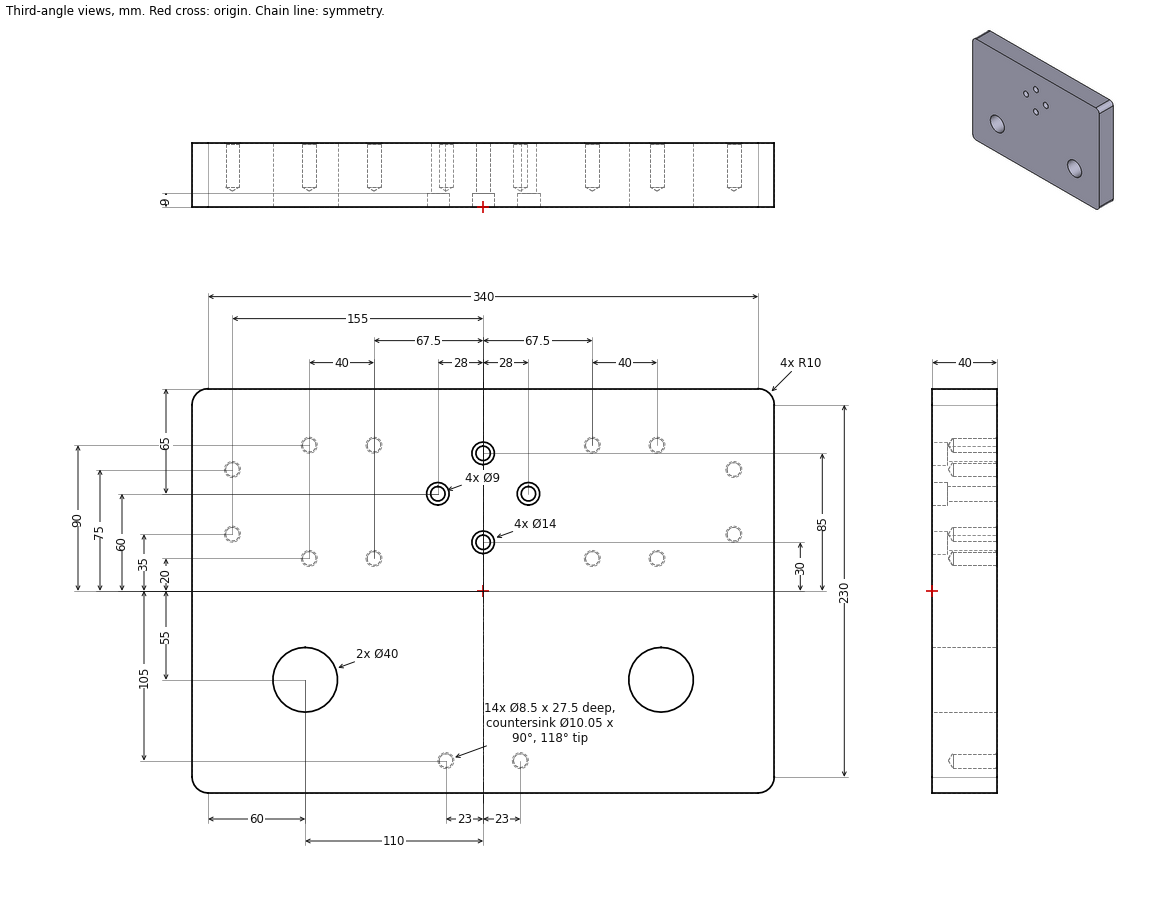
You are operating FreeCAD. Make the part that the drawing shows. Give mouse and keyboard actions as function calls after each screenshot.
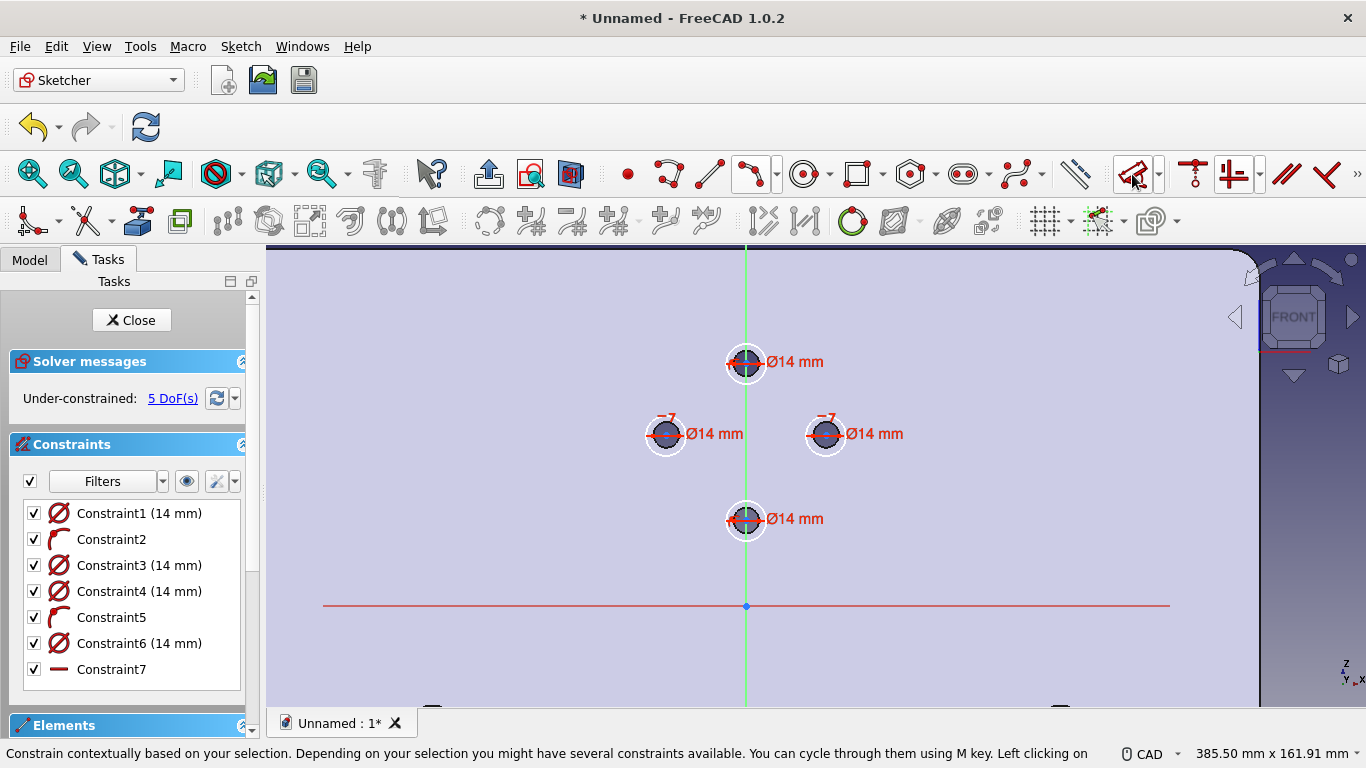
click(746, 521)
click(780, 564)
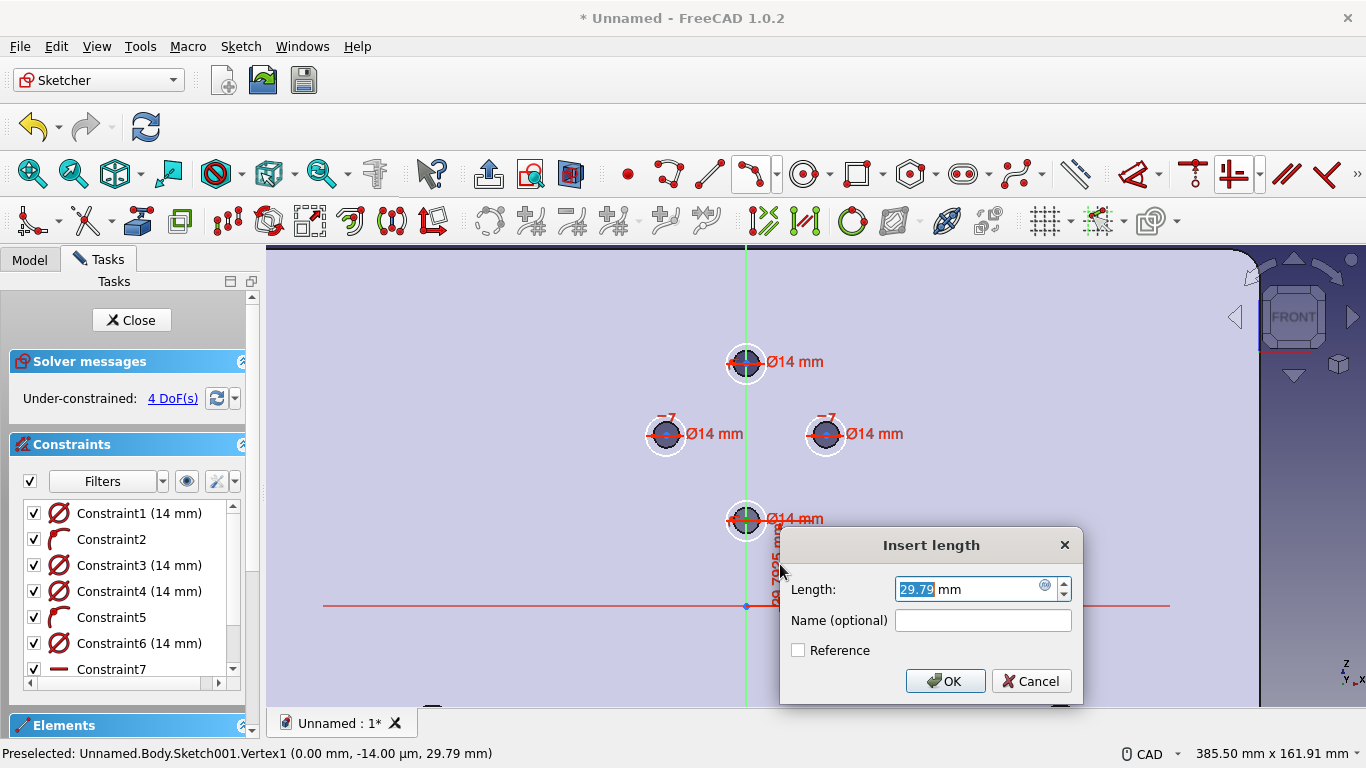
text(30)
key(Return)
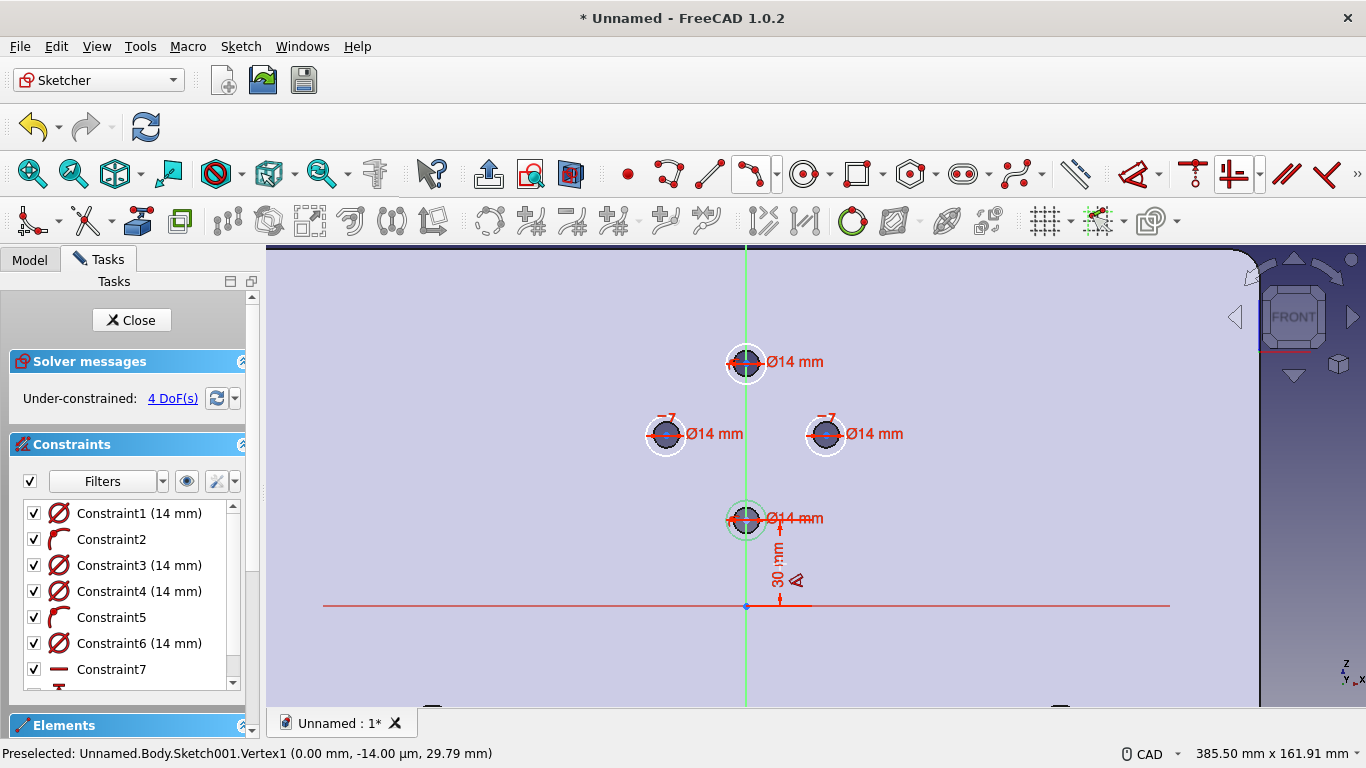
click(666, 436)
click(706, 640)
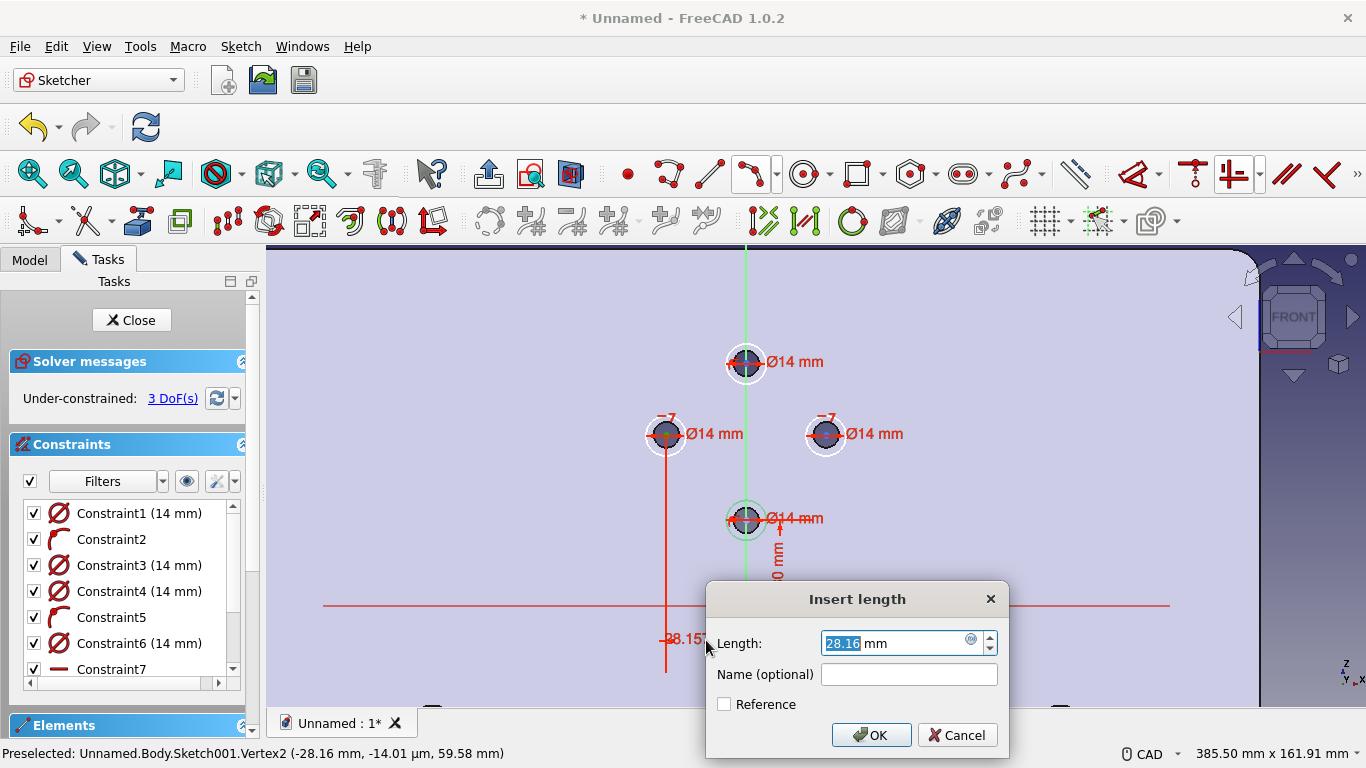
text(28)
key(Return)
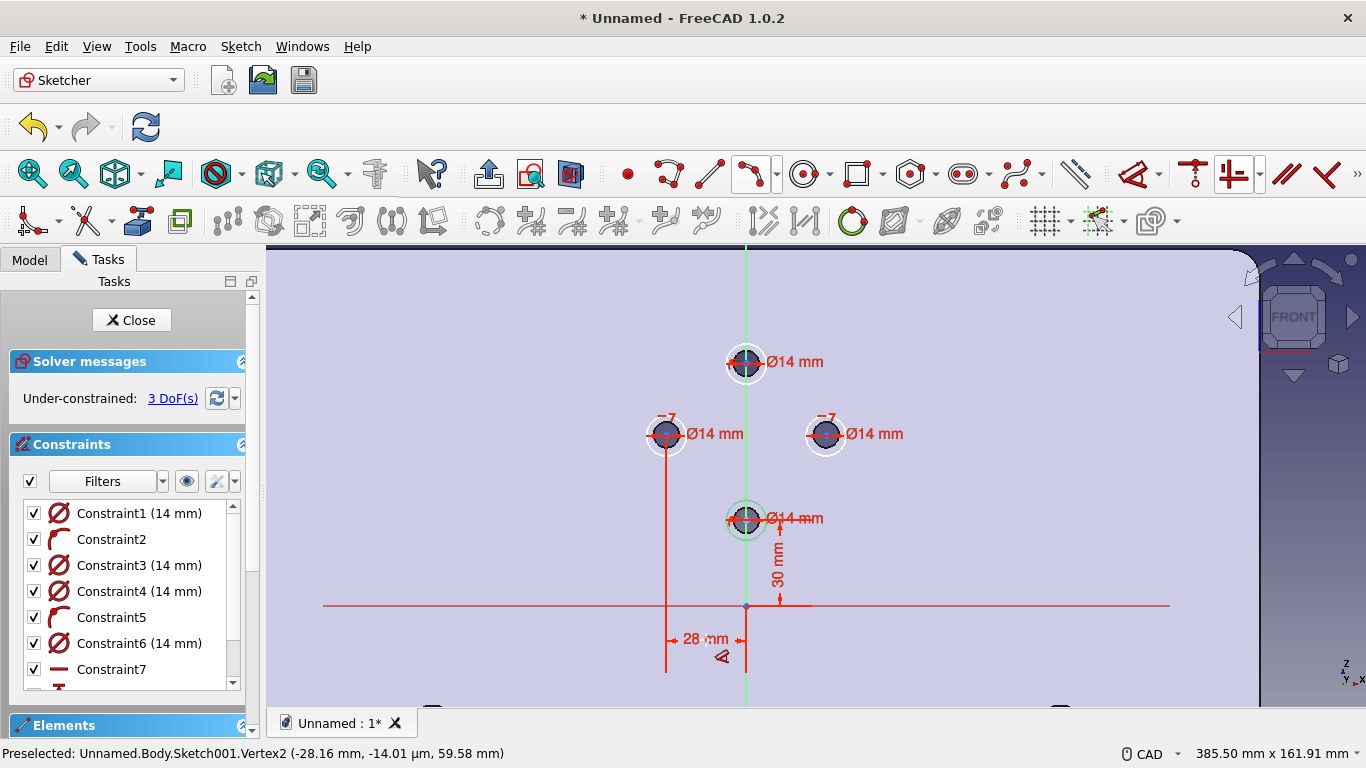
click(666, 436)
click(632, 521)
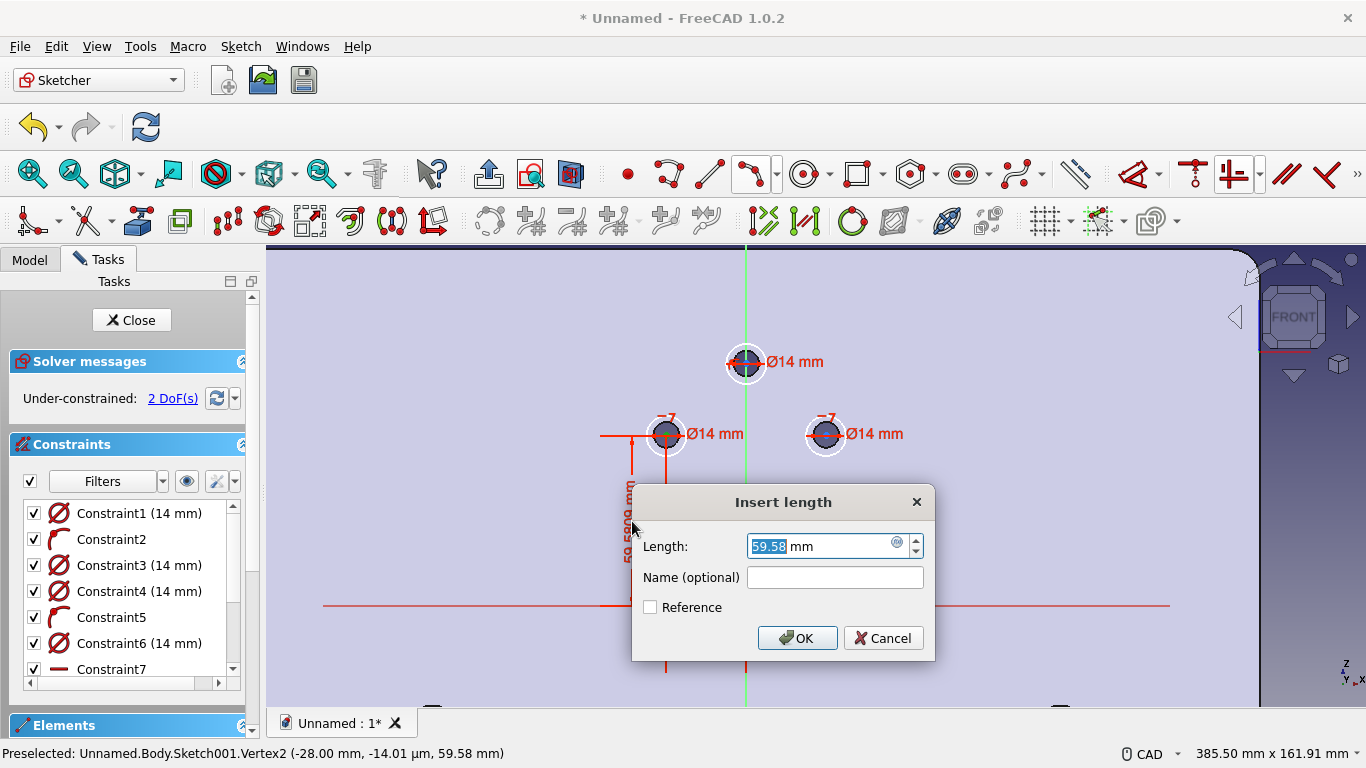
text(60)
key(Return)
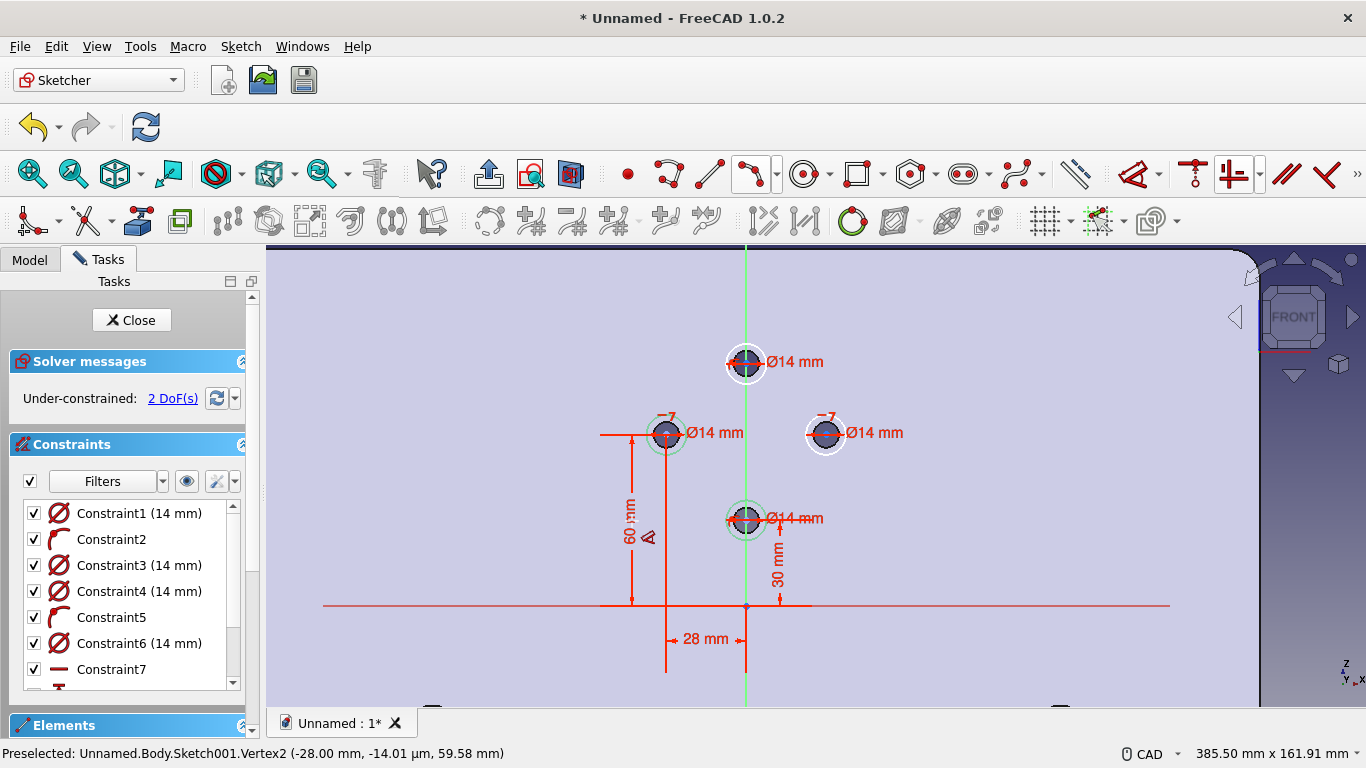
click(746, 364)
click(780, 485)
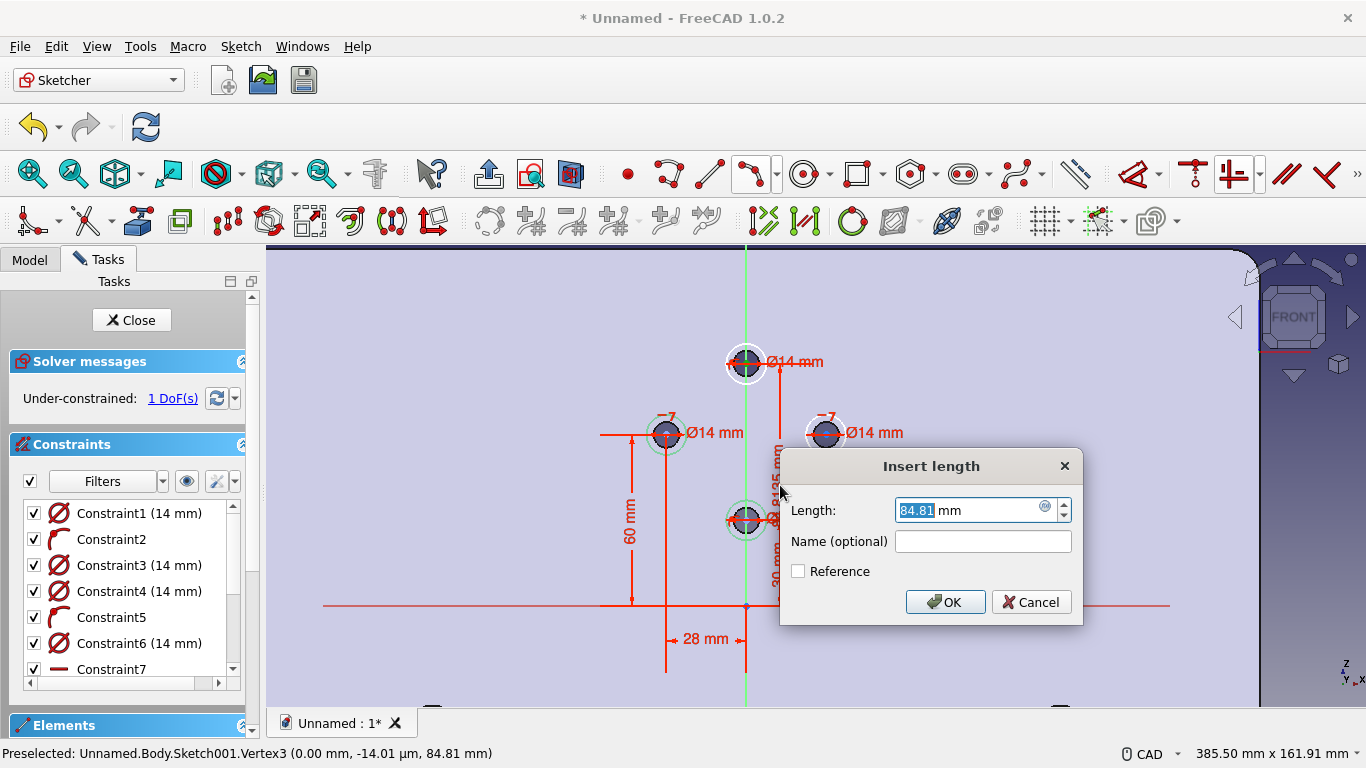
text(85)
key(Return)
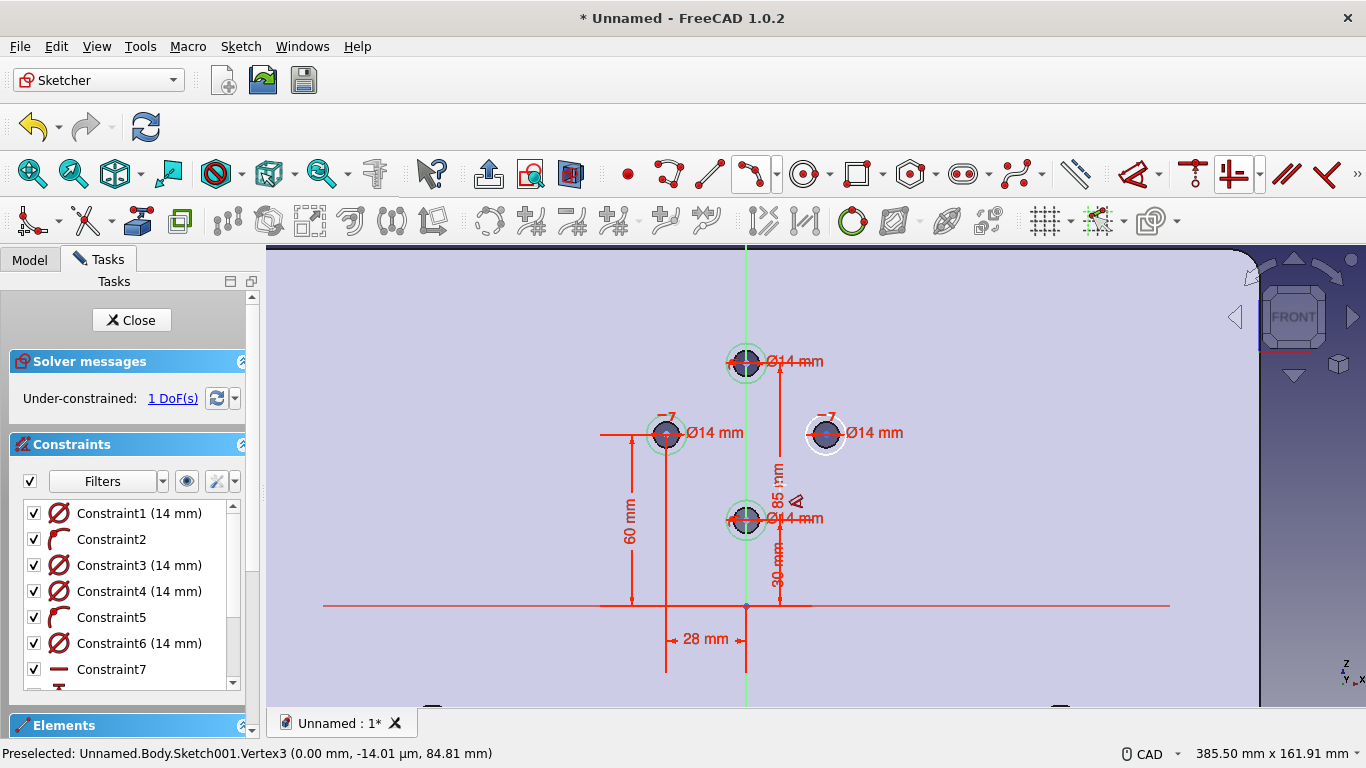
click(826, 435)
click(786, 640)